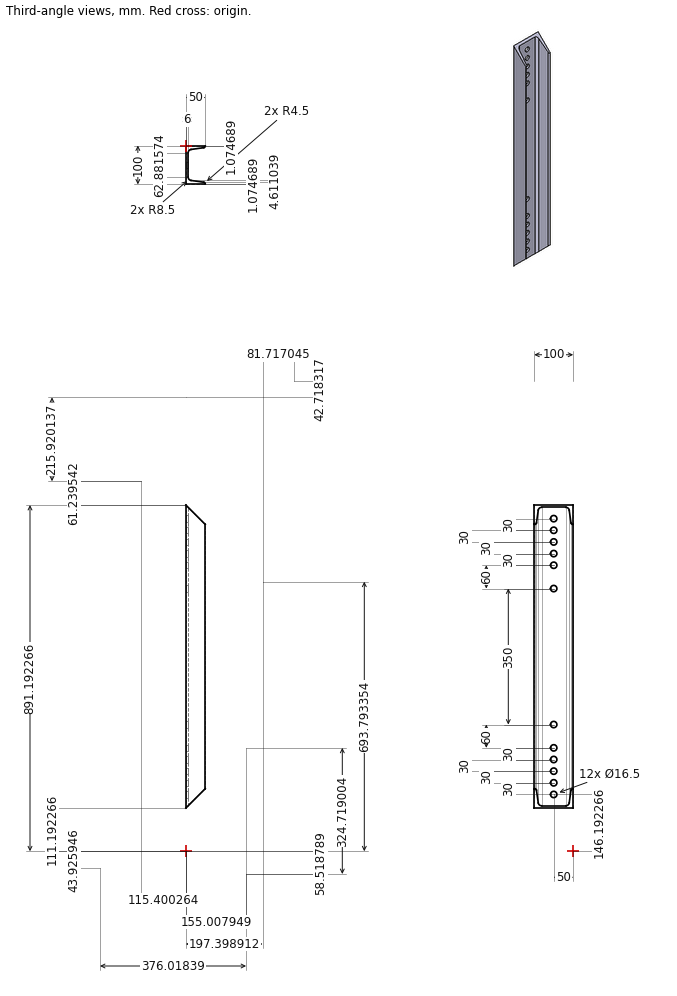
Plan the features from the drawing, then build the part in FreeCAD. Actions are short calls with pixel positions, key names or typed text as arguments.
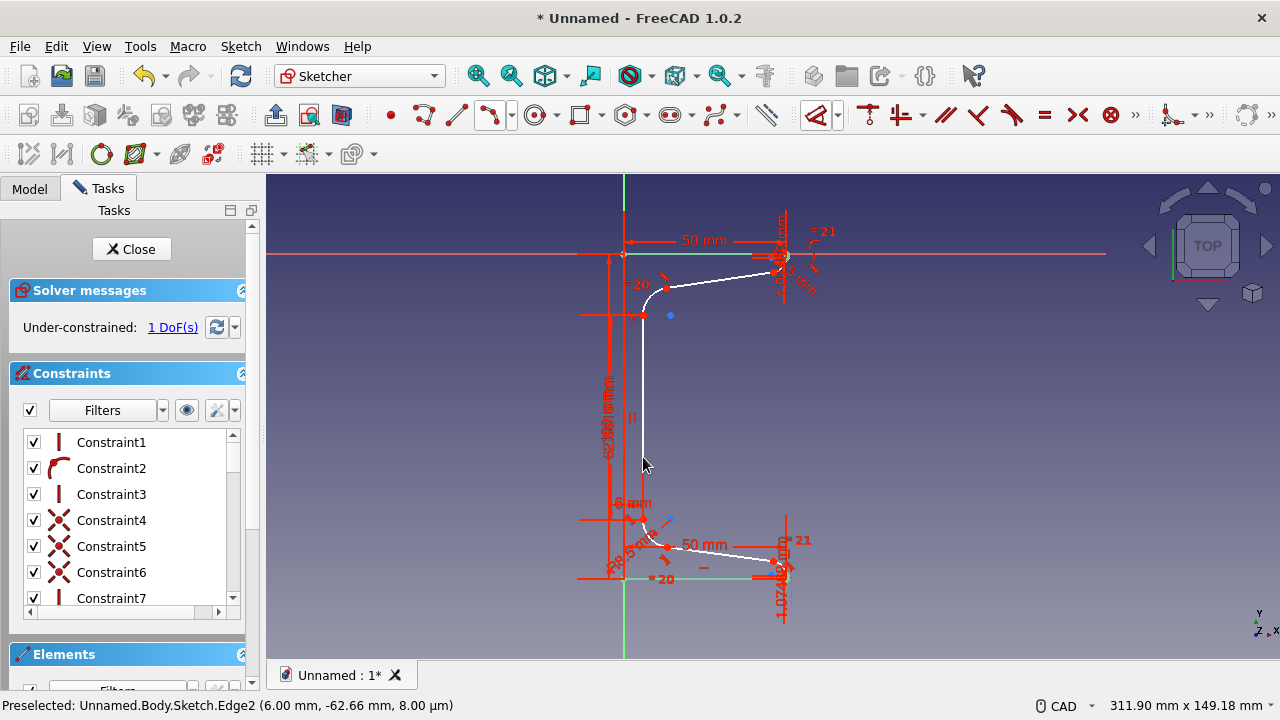
scroll(741, 557, up, 5)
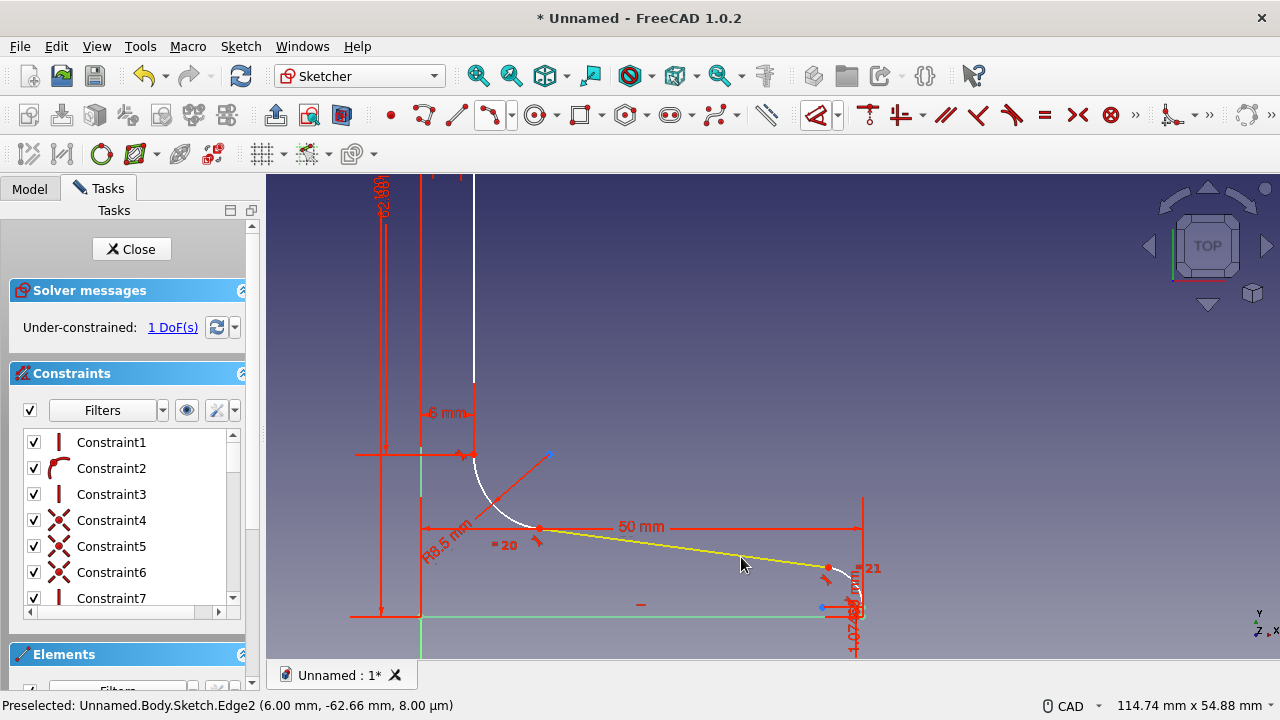
click(742, 556)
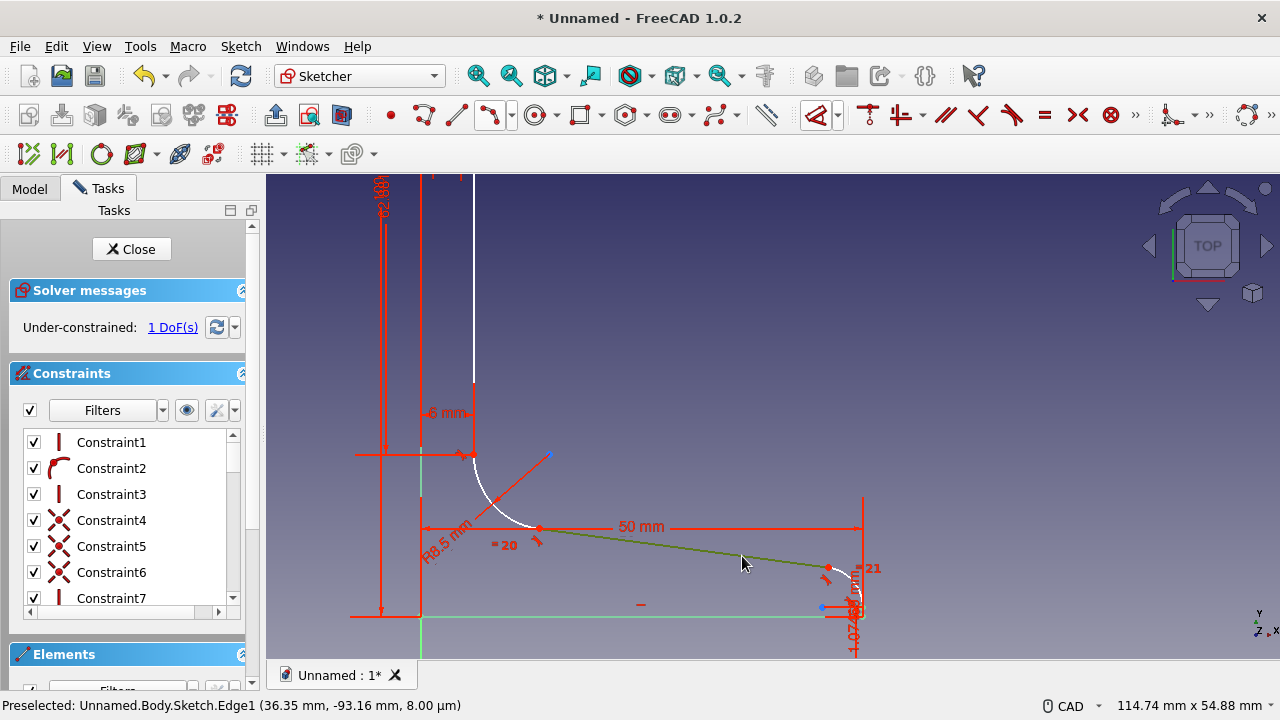
click(838, 116)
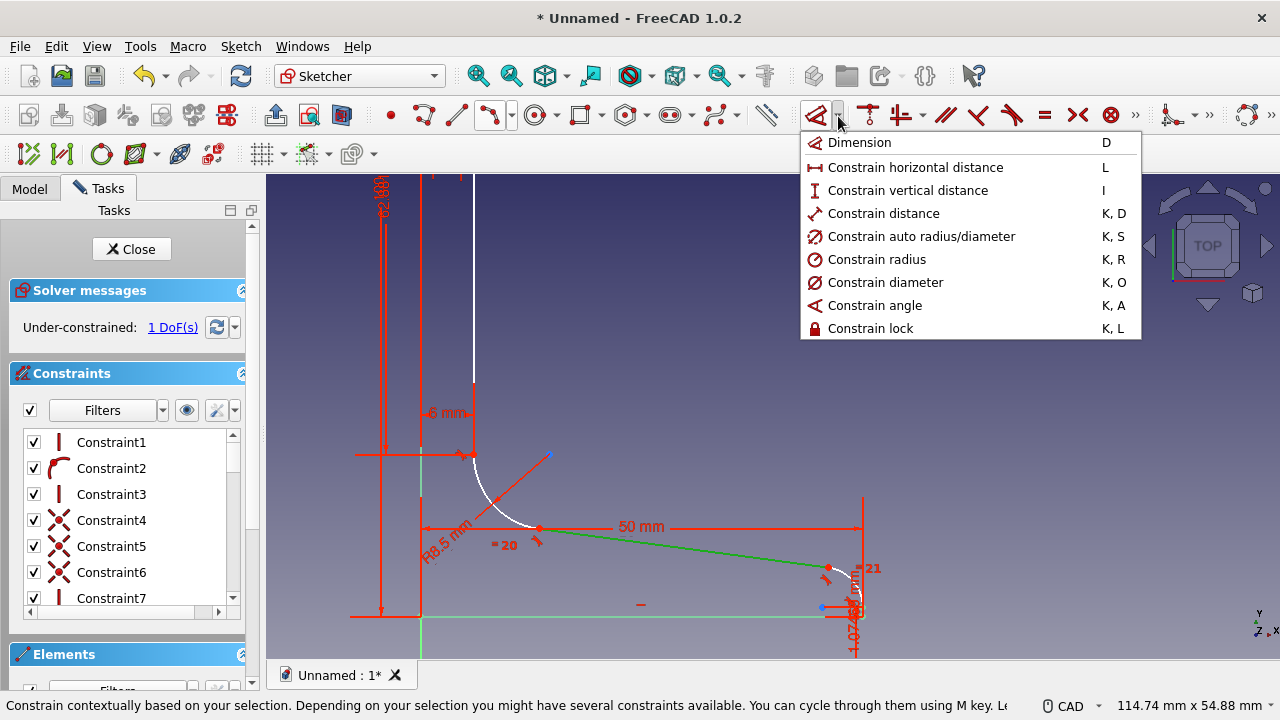
click(971, 190)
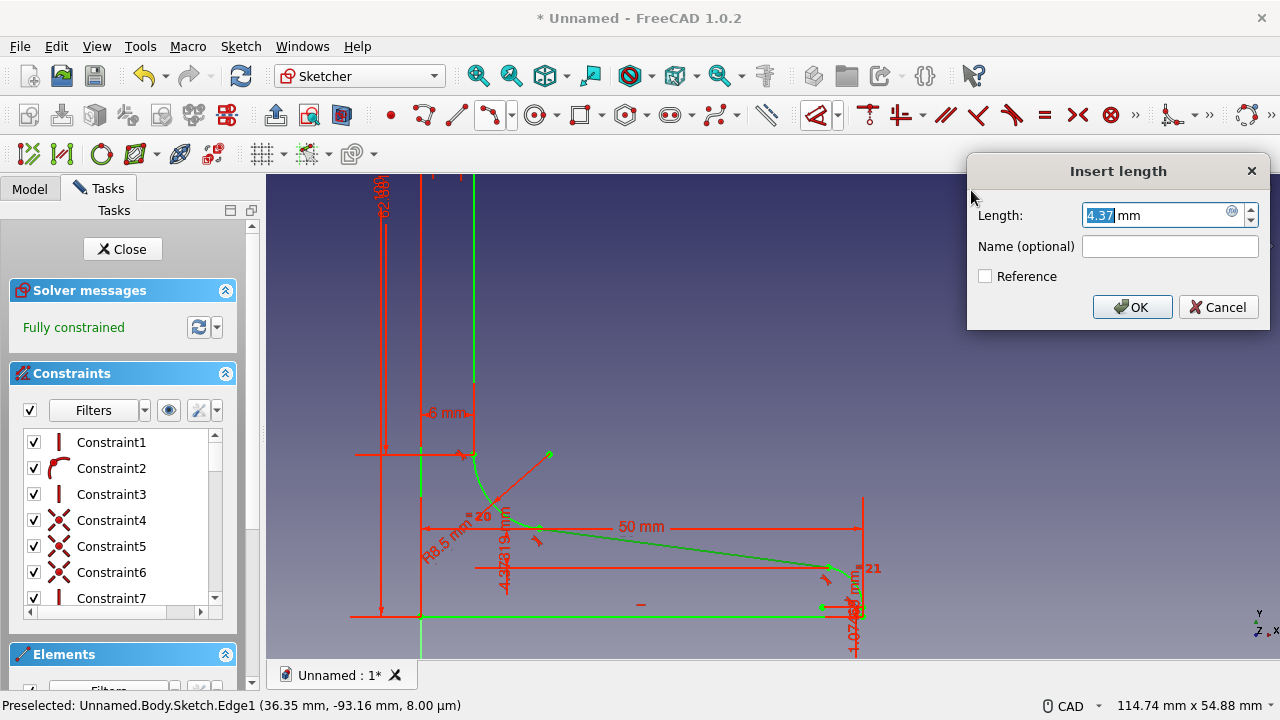
text(4.611039)
key(Return)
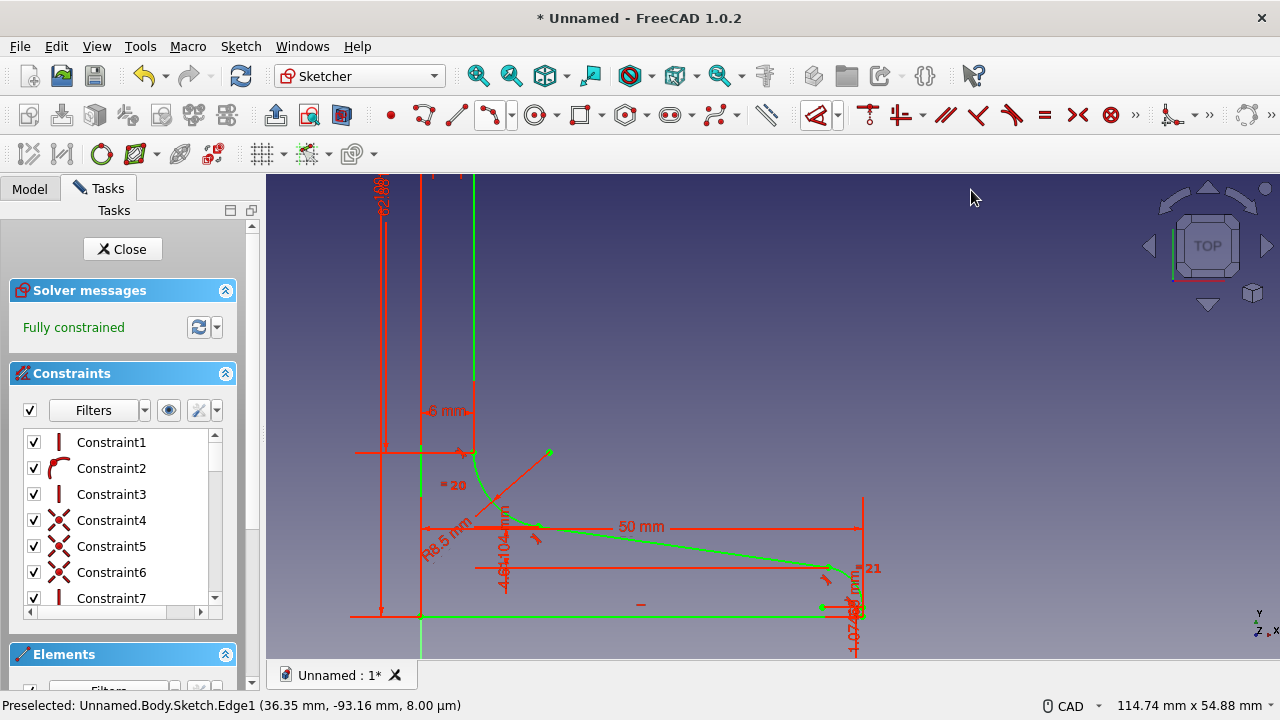
click(123, 249)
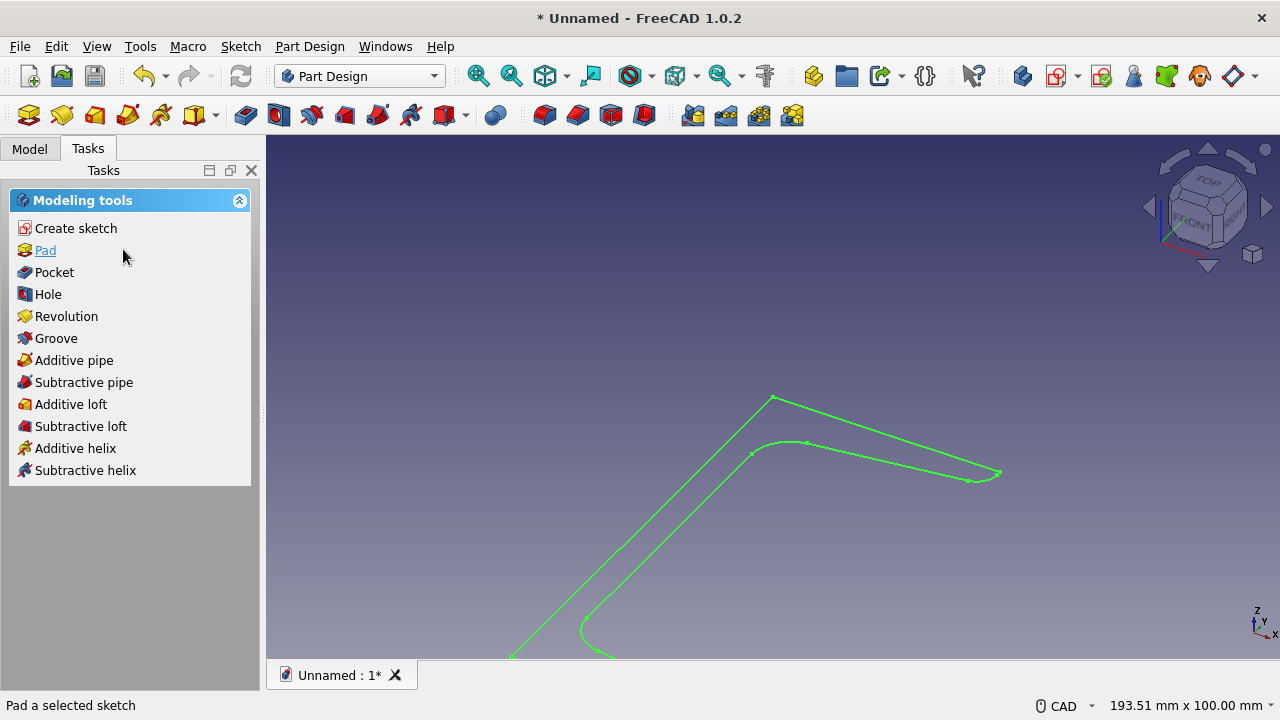
click(29, 116)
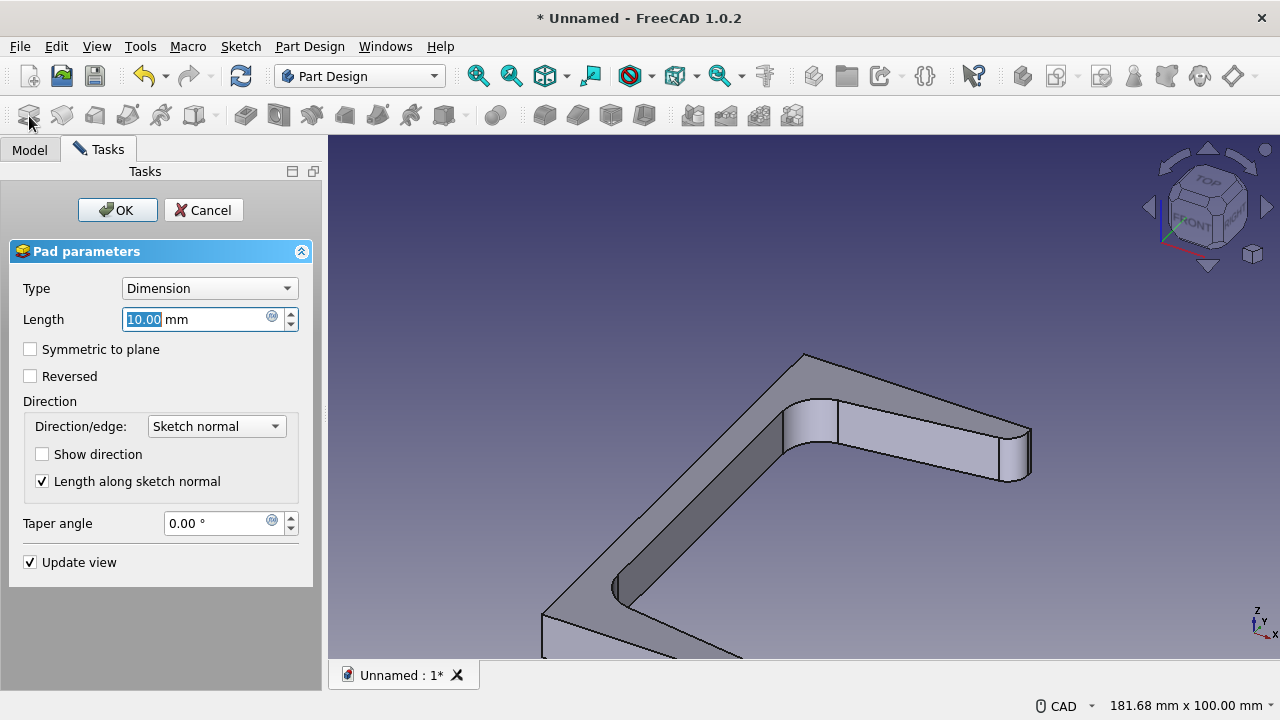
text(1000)
key(Tab)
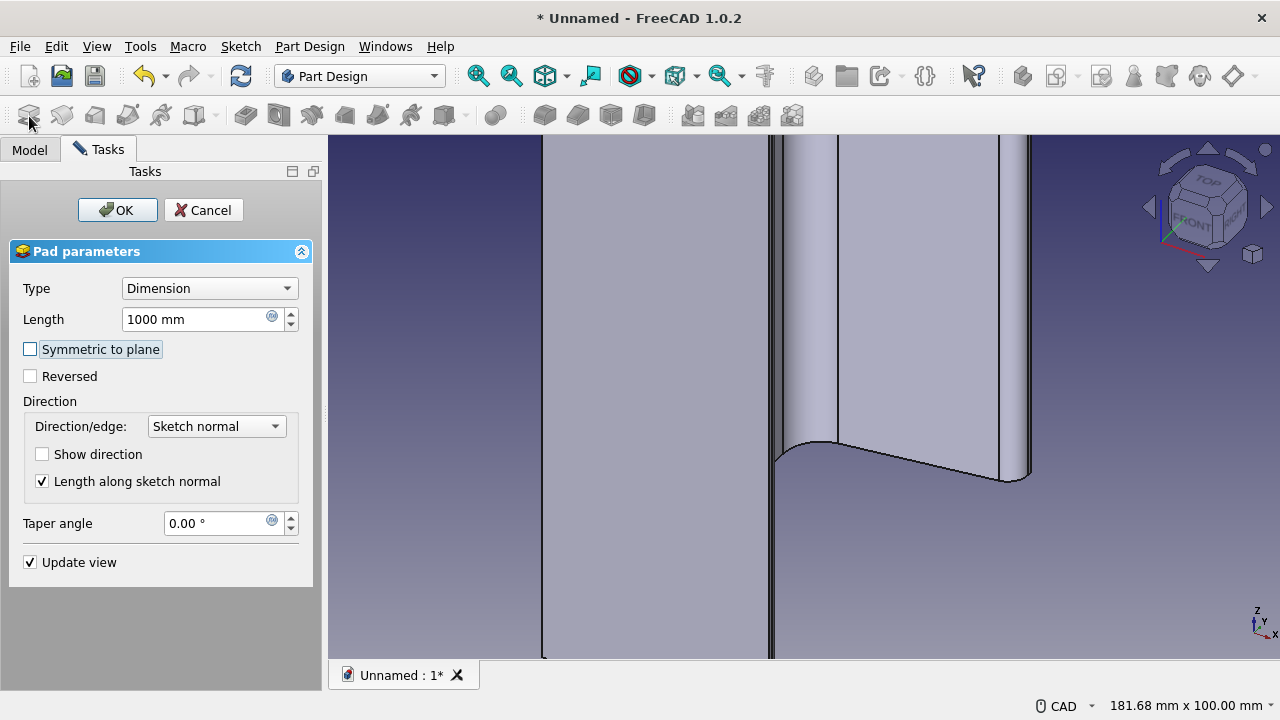
click(118, 210)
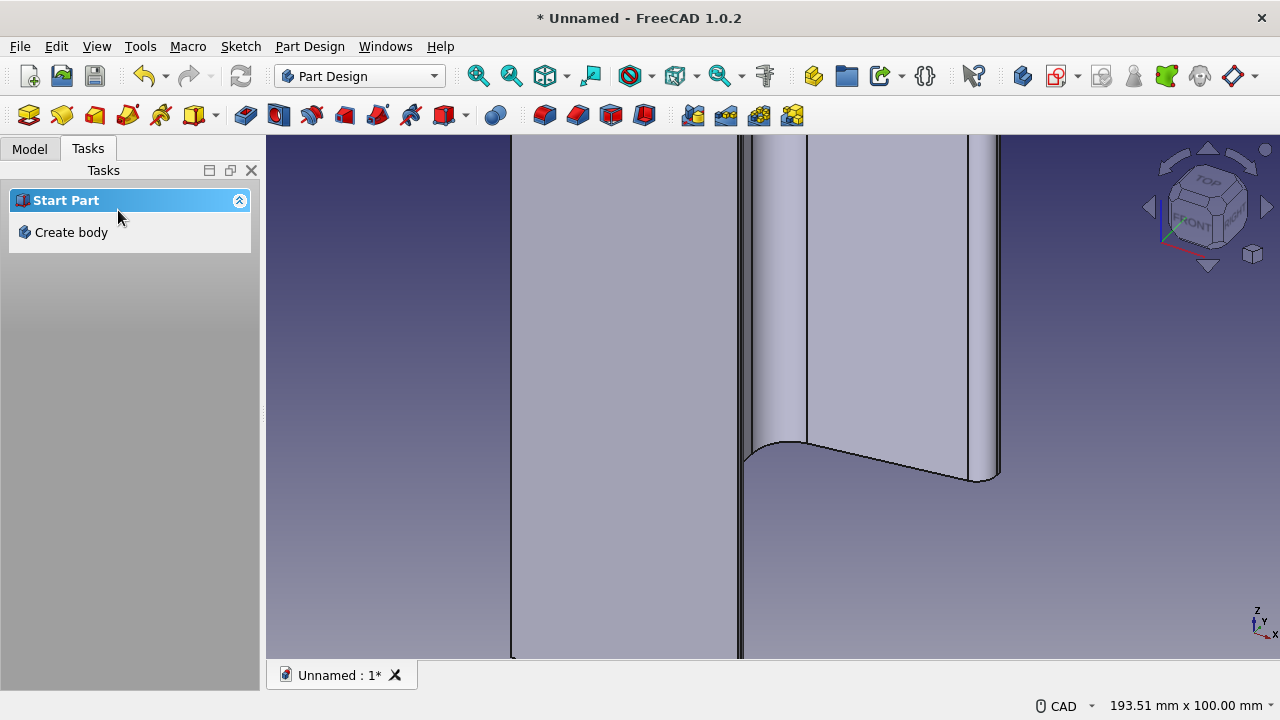
click(479, 76)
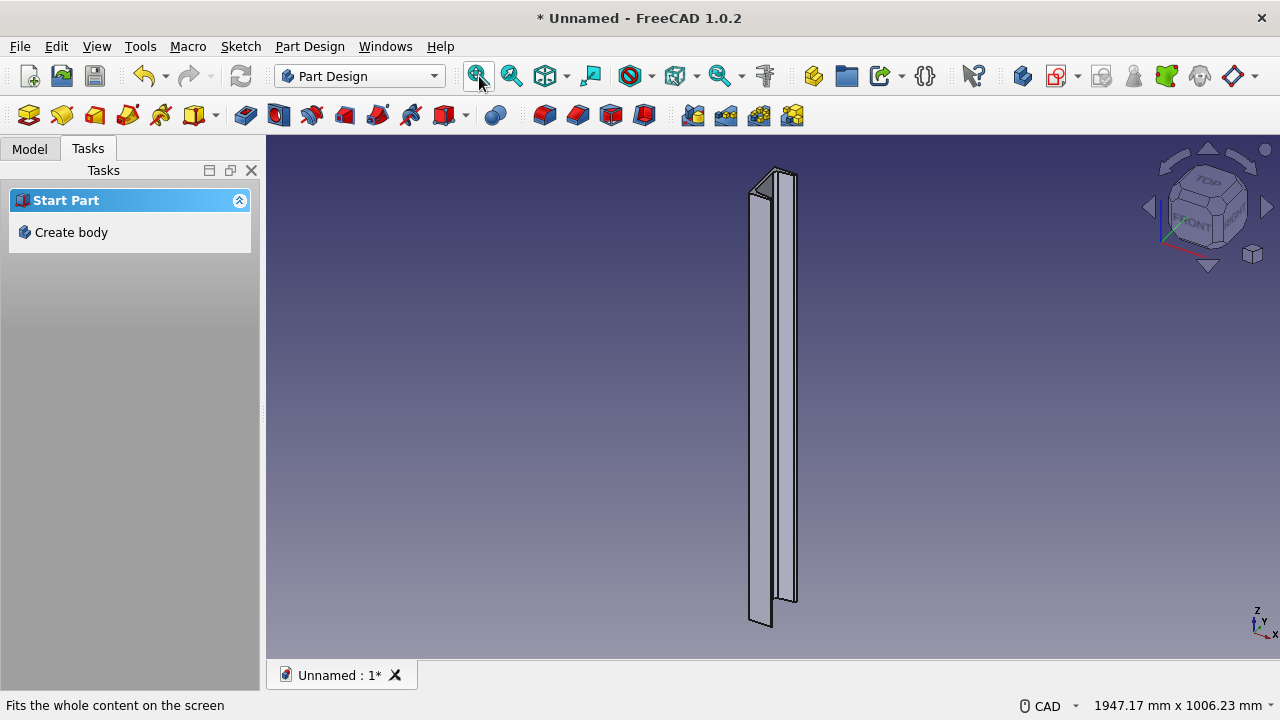
key(4)